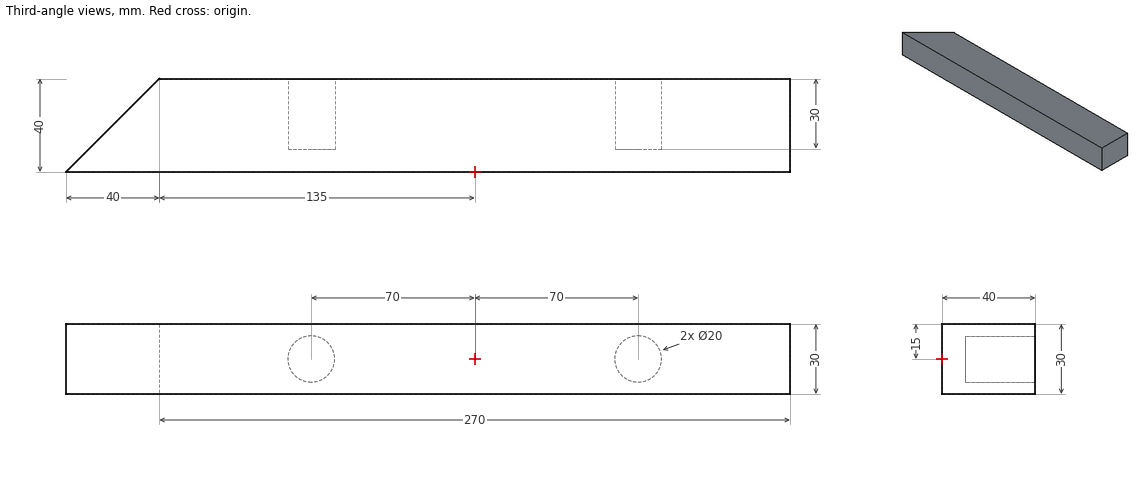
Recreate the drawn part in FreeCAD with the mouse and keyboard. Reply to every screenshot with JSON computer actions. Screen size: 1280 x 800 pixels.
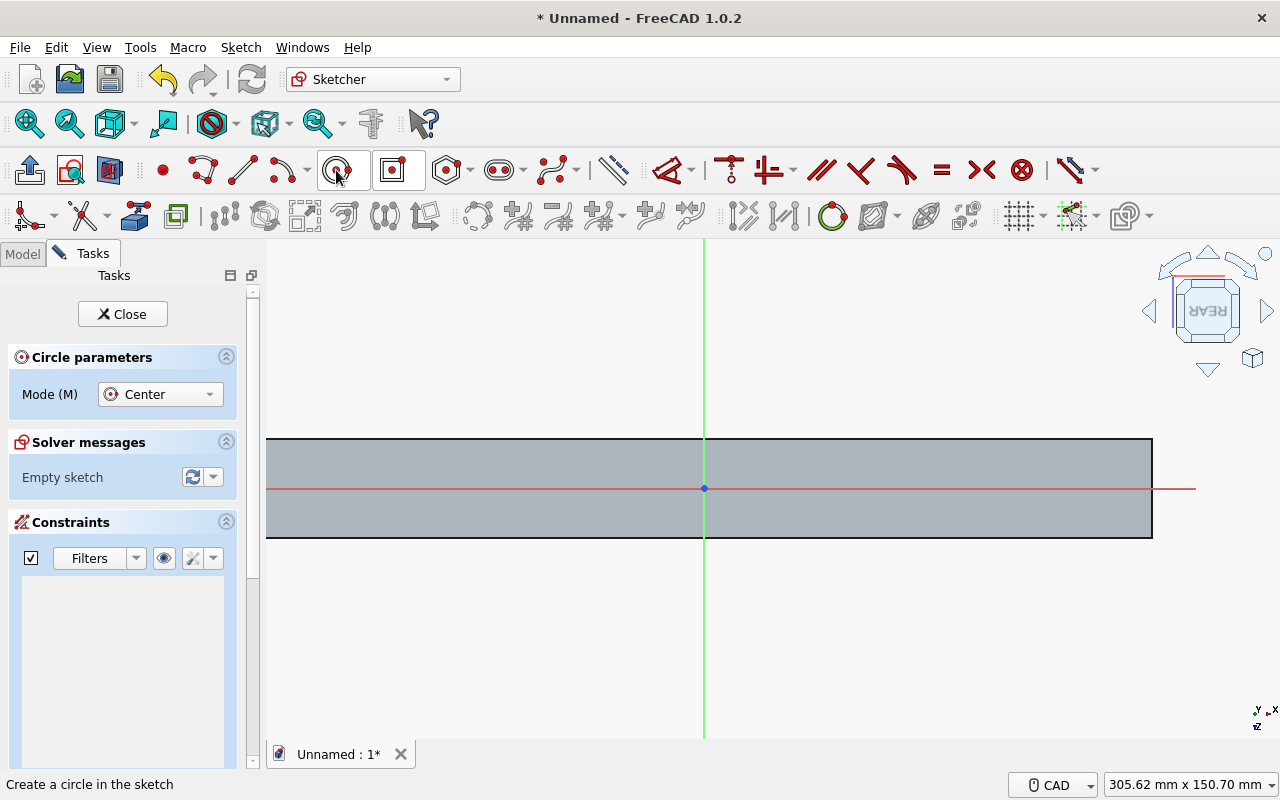
{"action": "left_click", "coordinate": [937, 489]}
{"action": "mouse_move", "coordinate": [960, 465]}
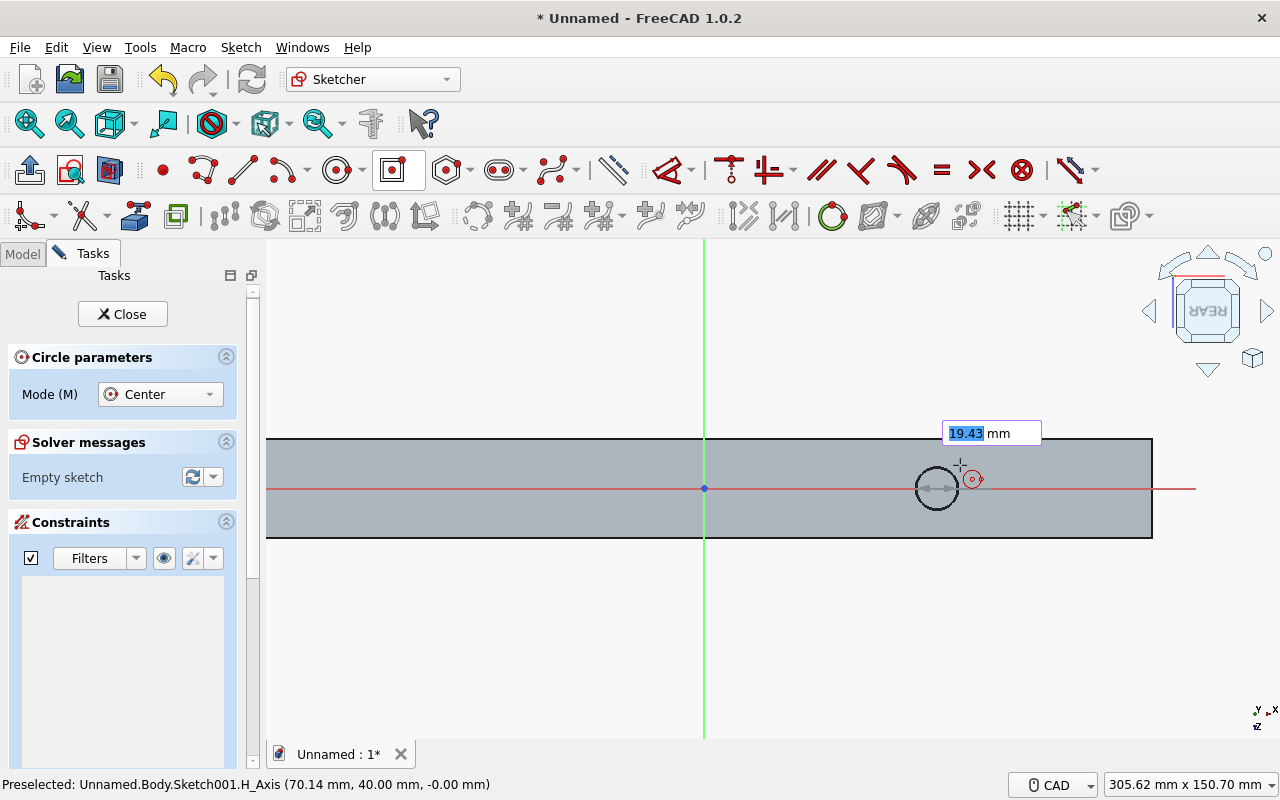
{"action": "type", "text": "20"}
{"action": "key", "text": "Return"}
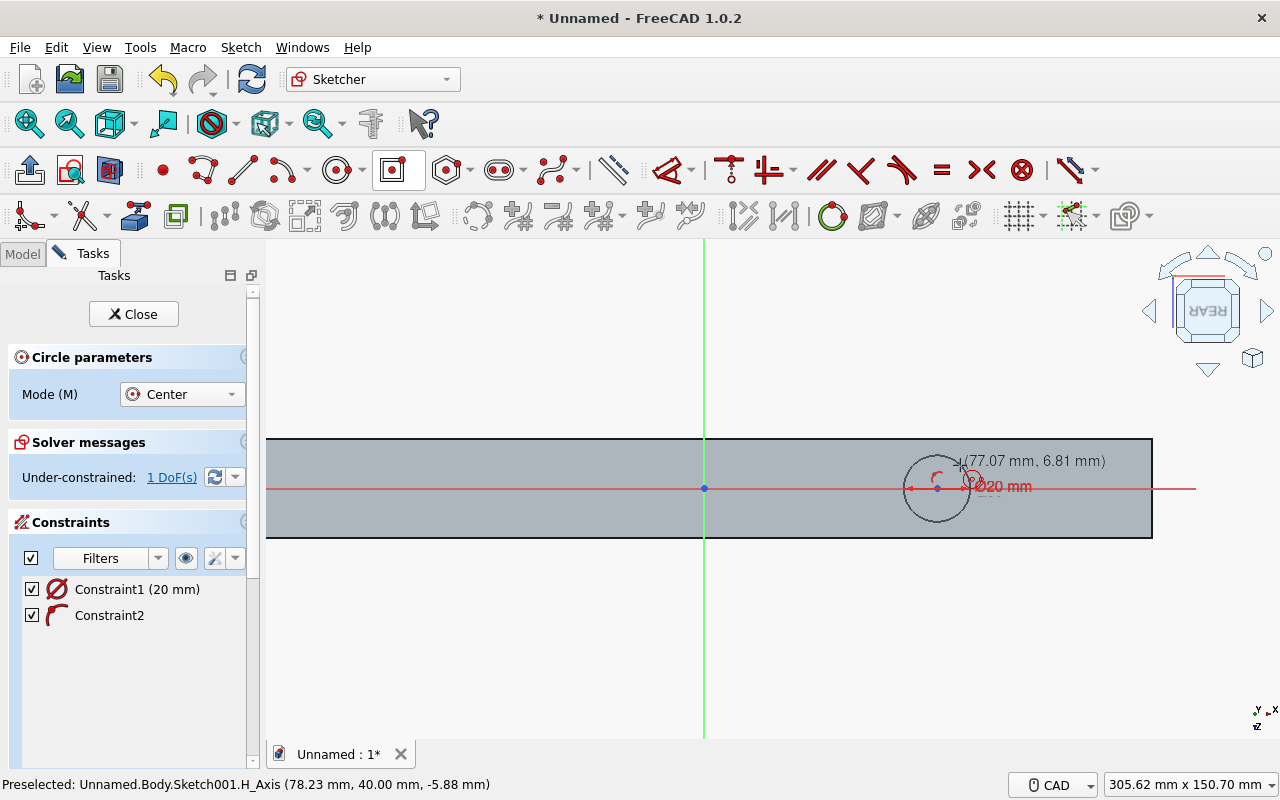
{"action": "left_click", "coordinate": [472, 489]}
{"action": "mouse_move", "coordinate": [495, 465]}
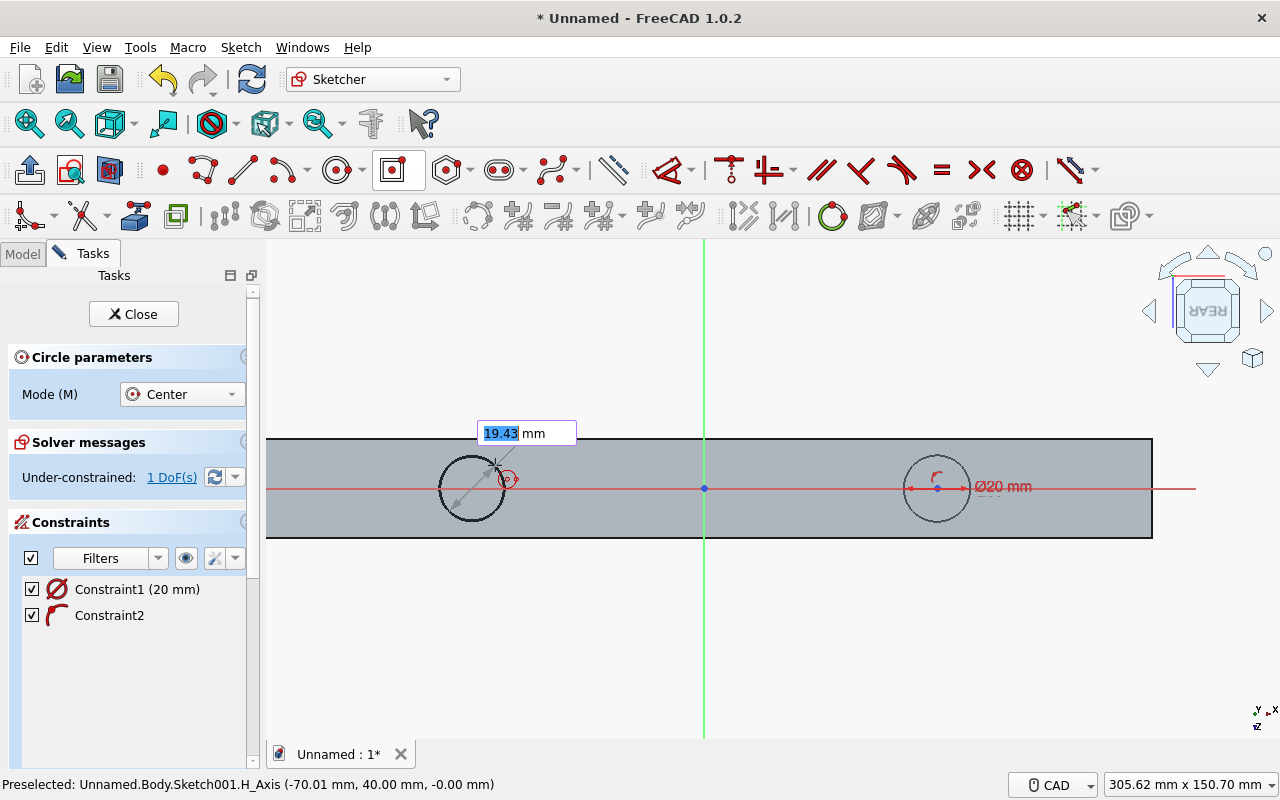
{"action": "type", "text": "20"}
{"action": "key", "text": "Return"}
{"action": "key", "text": "Escape"}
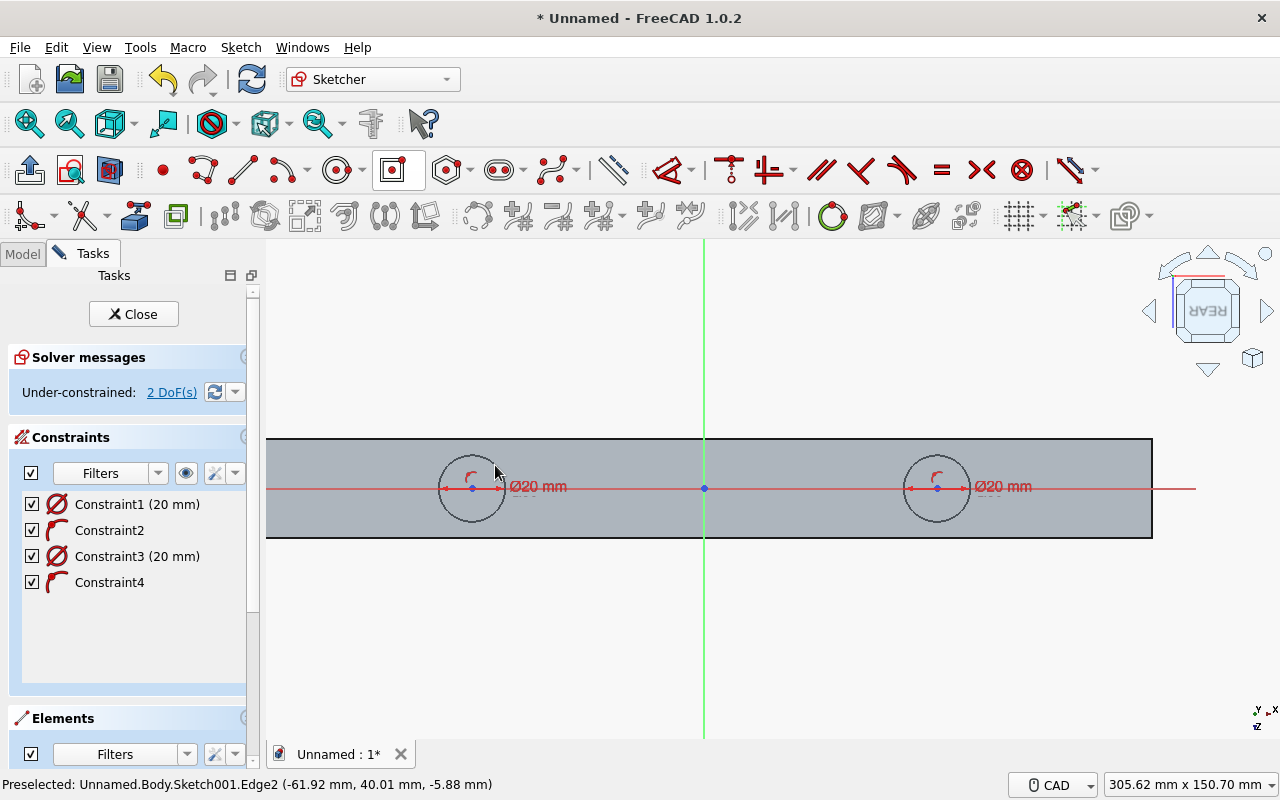
{"action": "left_click", "coordinate": [668, 170]}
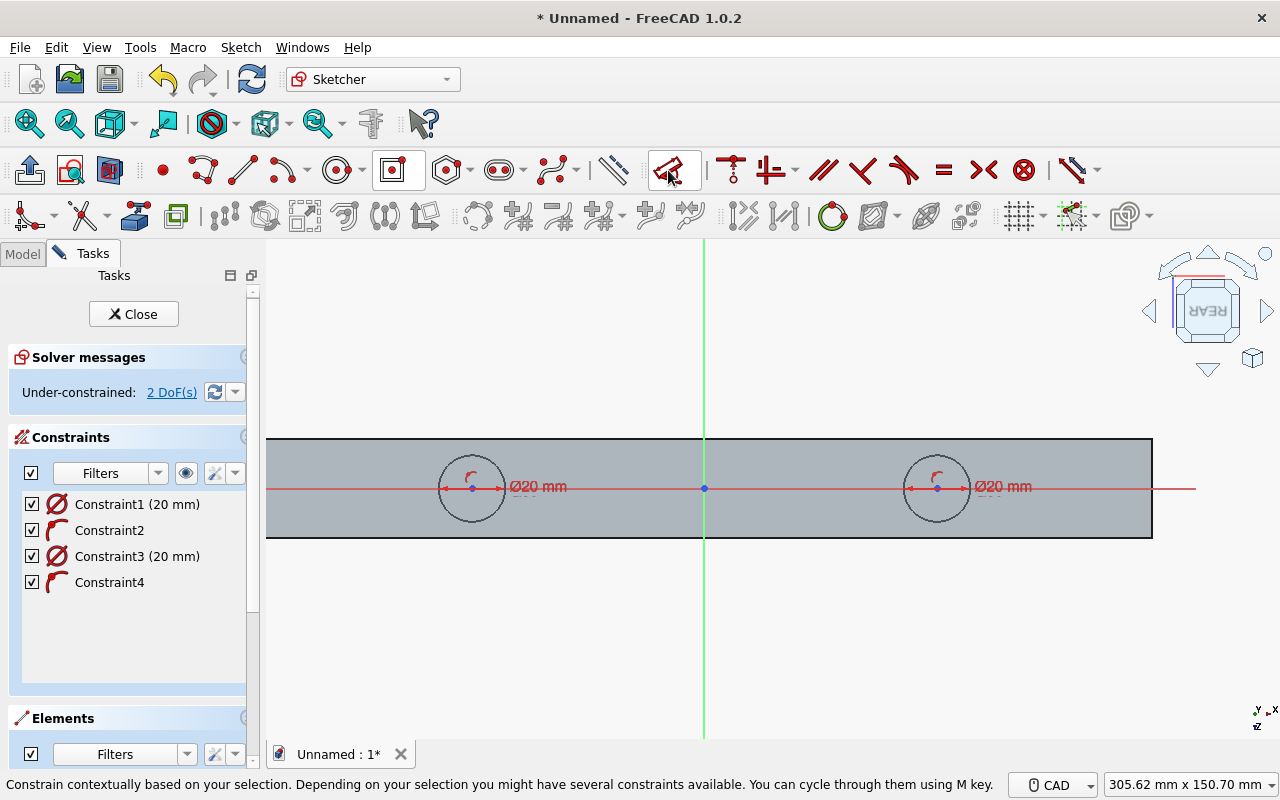
{"action": "left_click", "coordinate": [937, 489]}
{"action": "left_click", "coordinate": [821, 523]}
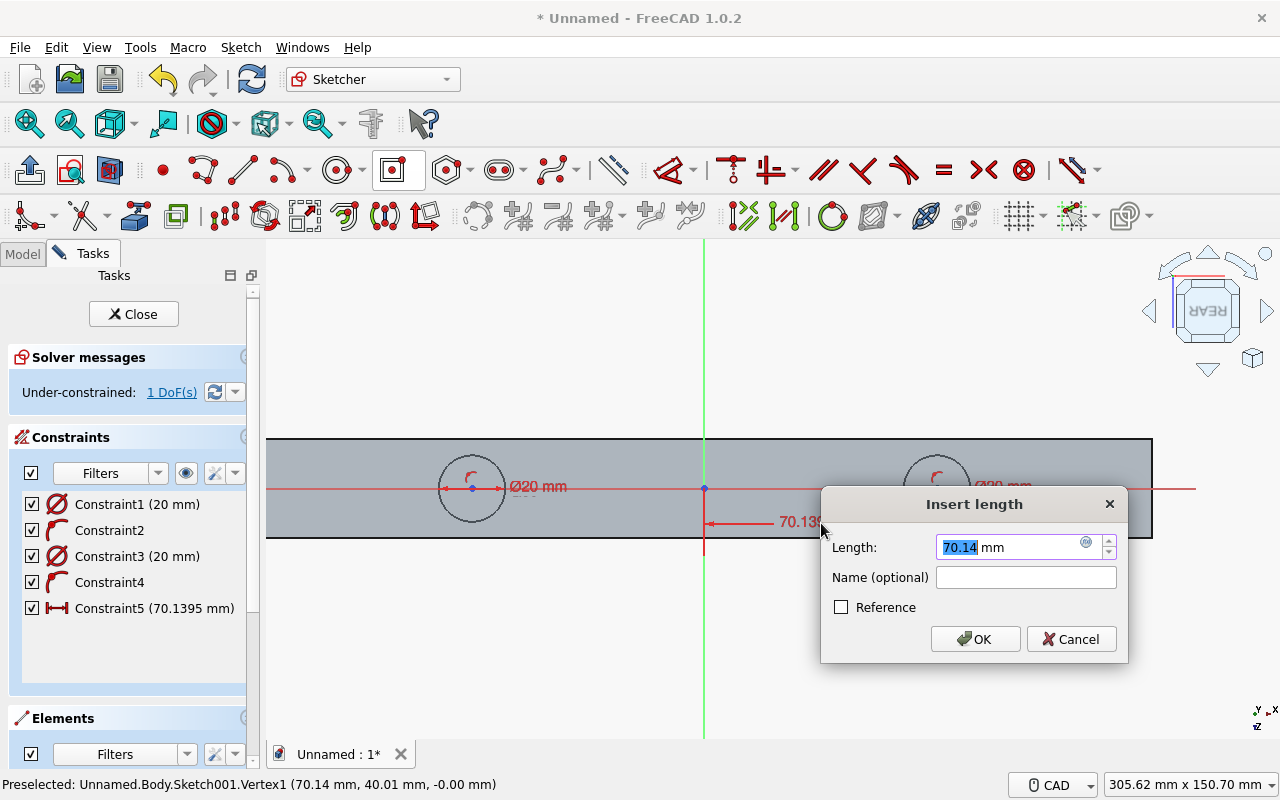
{"action": "type", "text": "70"}
{"action": "key", "text": "Return"}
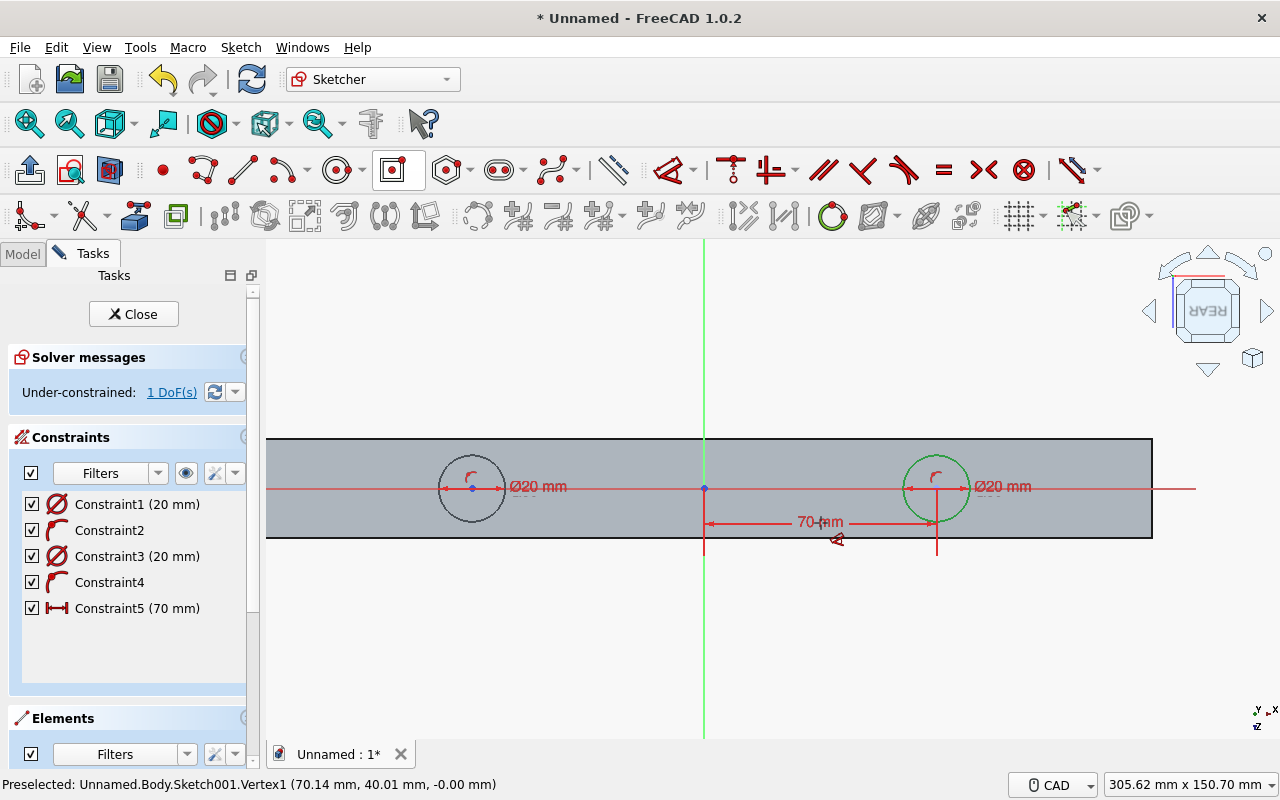
{"action": "left_click", "coordinate": [472, 489]}
{"action": "left_click", "coordinate": [588, 523]}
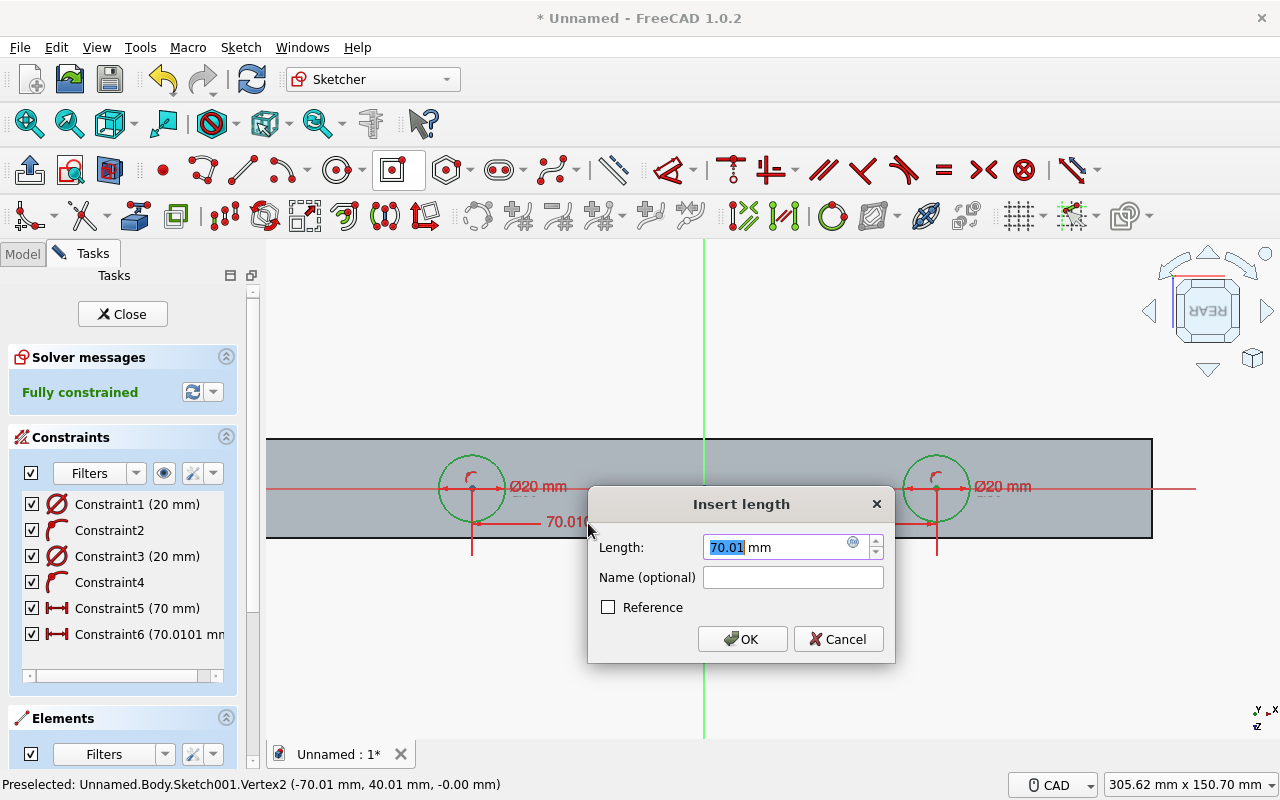
{"action": "type", "text": "70"}
{"action": "key", "text": "Return"}
{"action": "key", "text": "Escape"}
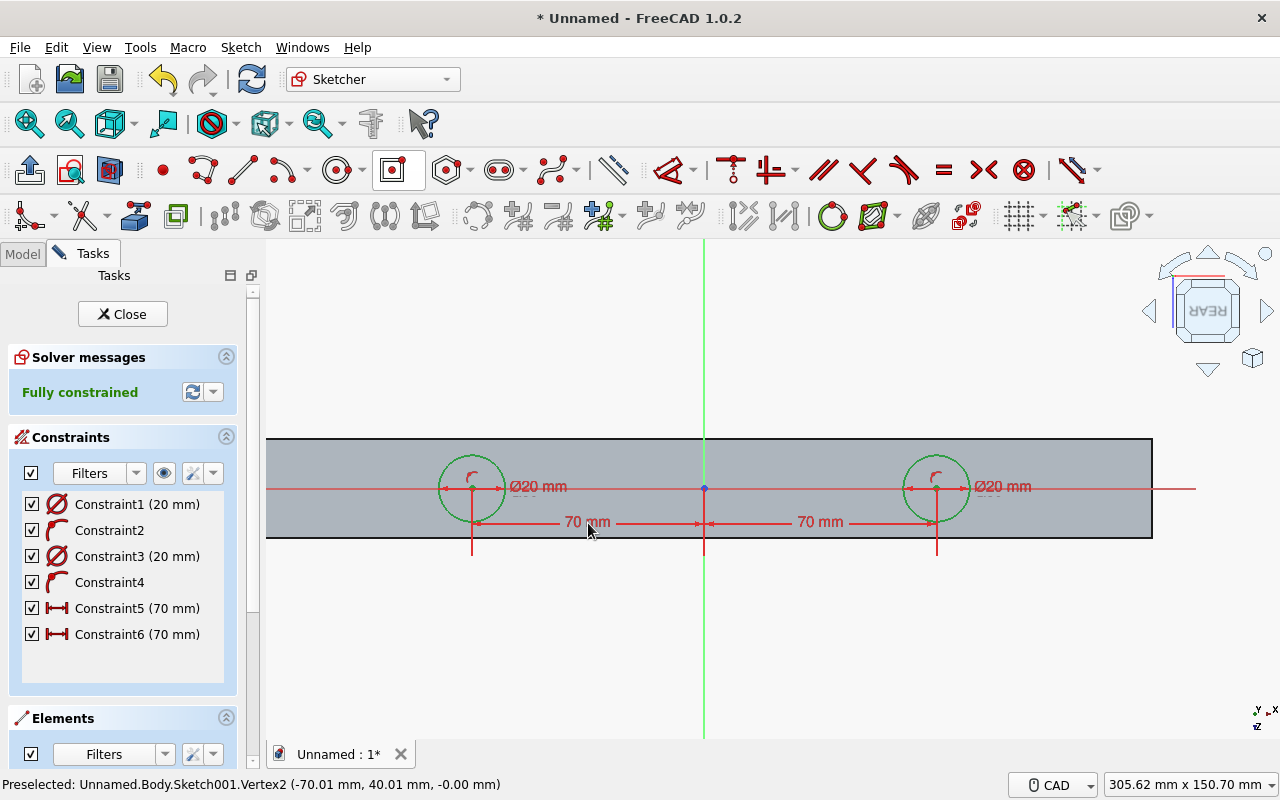
{"action": "left_click", "coordinate": [123, 314]}